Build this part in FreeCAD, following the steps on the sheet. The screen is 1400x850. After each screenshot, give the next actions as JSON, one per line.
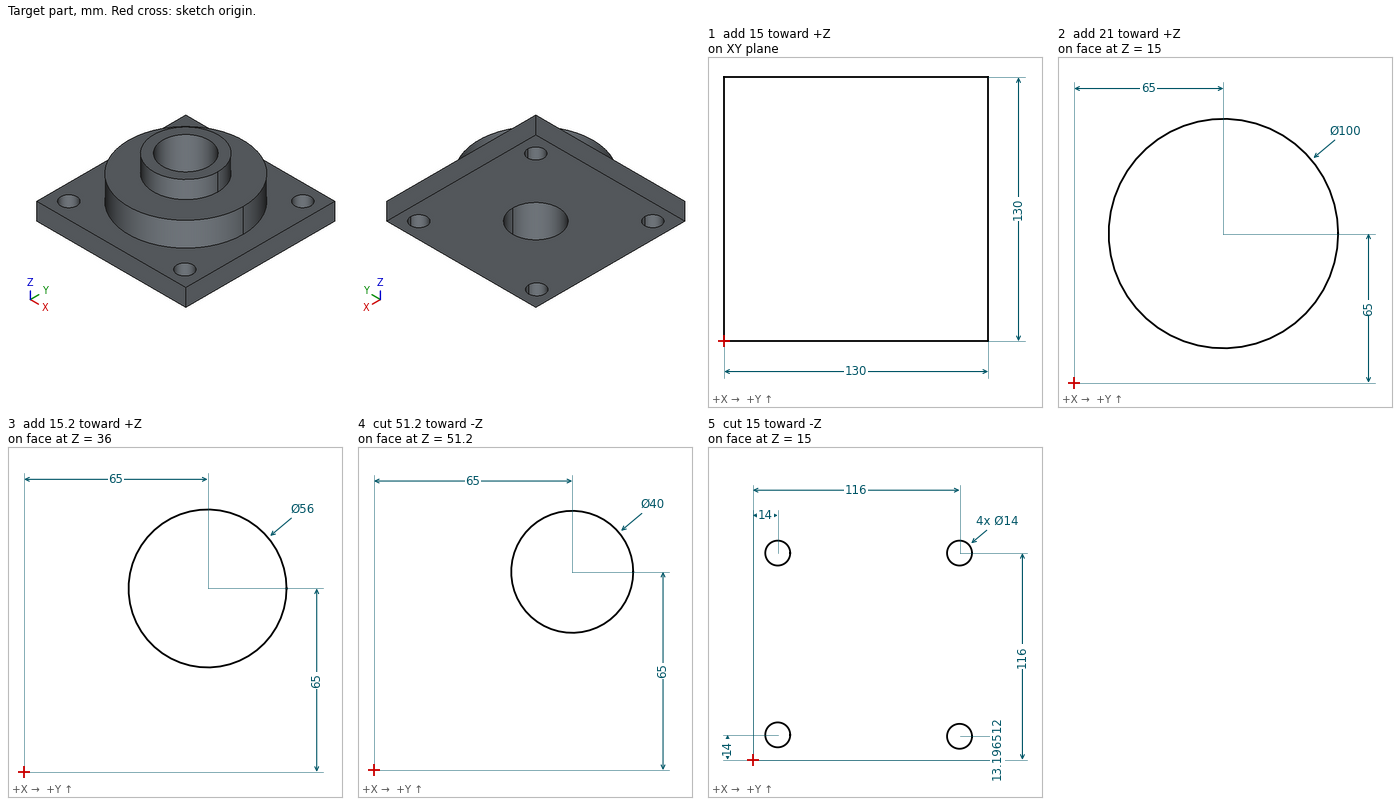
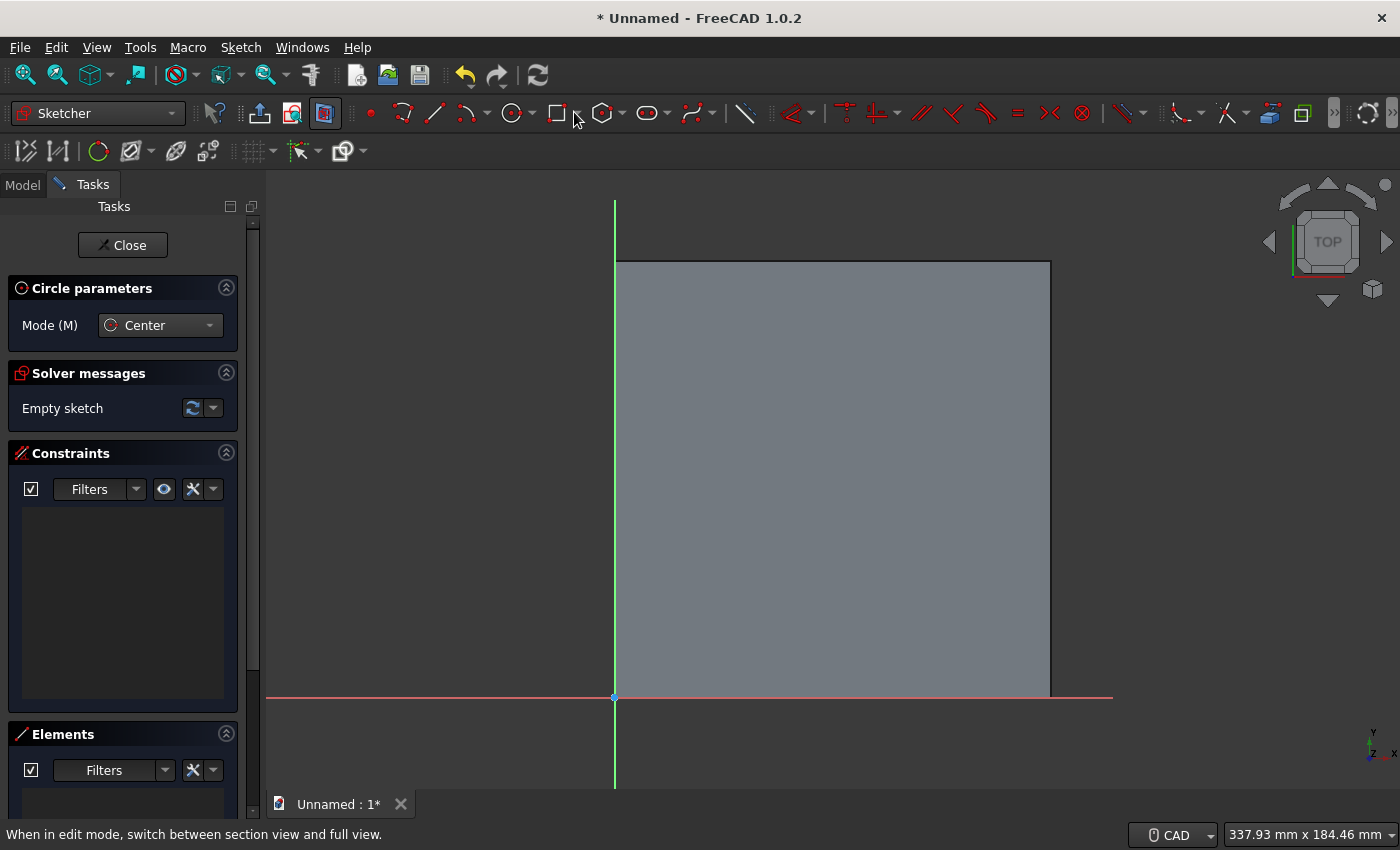
{"action": "left_click", "coordinate": [833, 480]}
{"action": "mouse_move", "coordinate": [952, 361]}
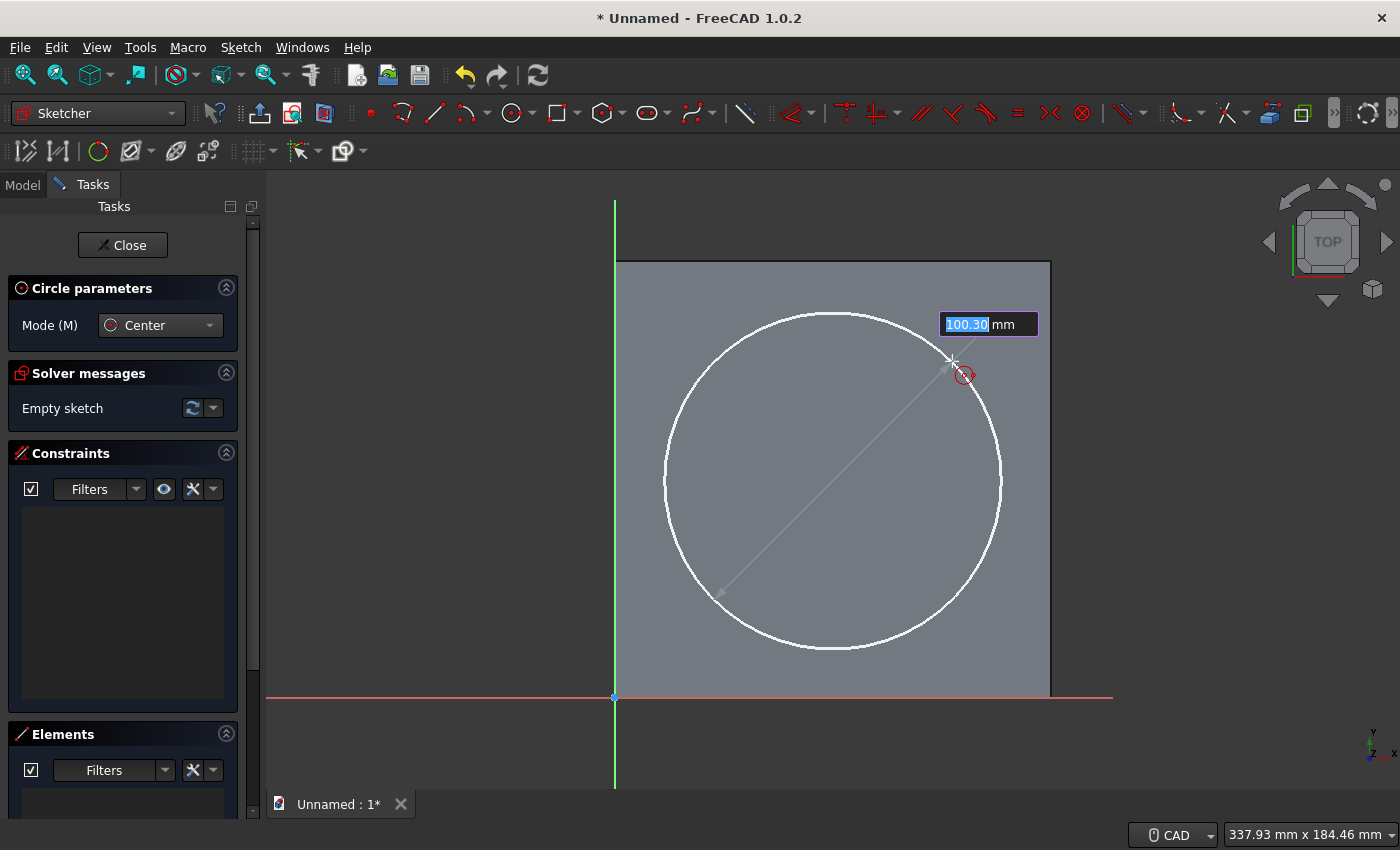
{"action": "type", "text": "100"}
{"action": "key", "text": "Return"}
{"action": "key", "text": "Escape"}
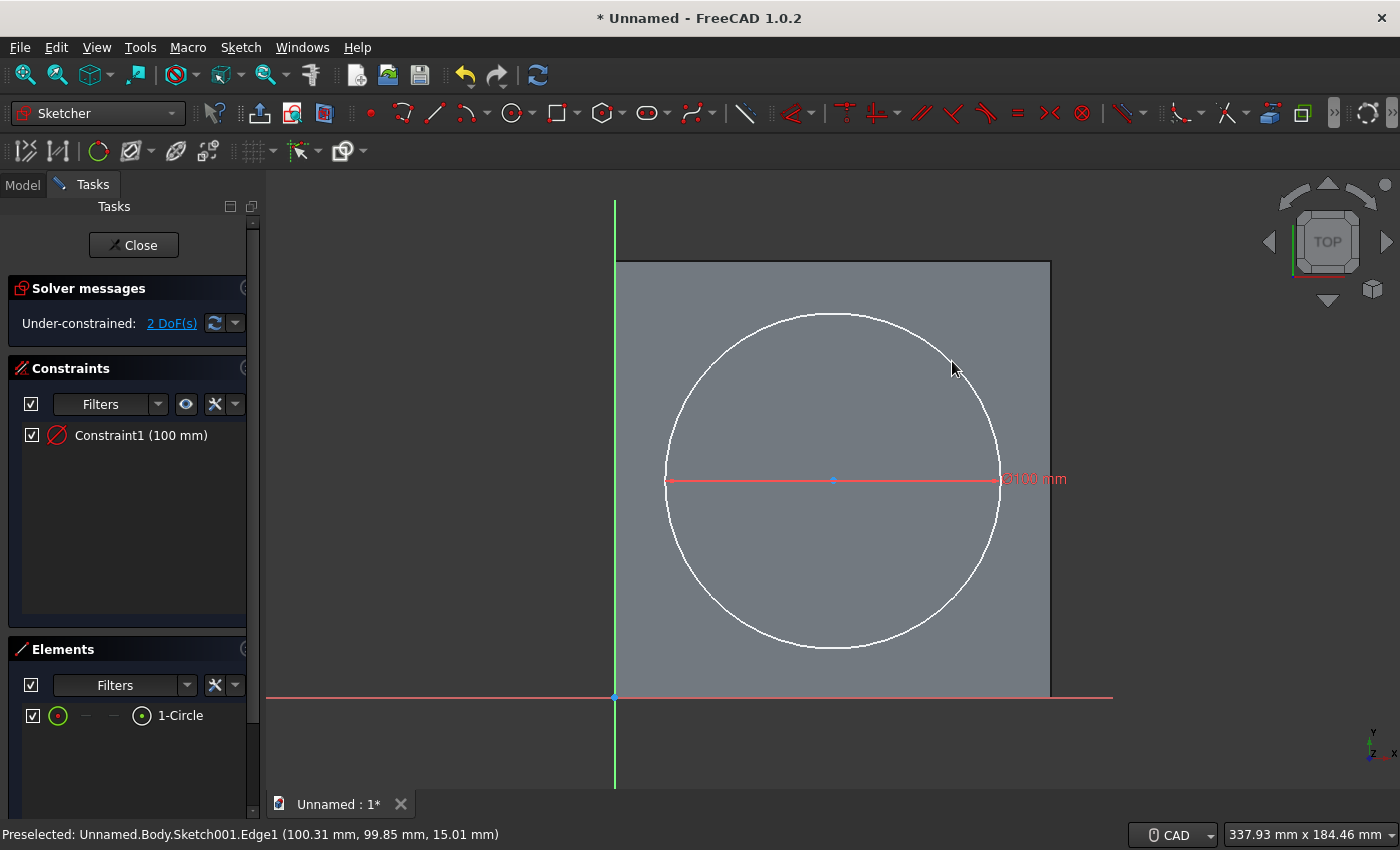
{"action": "key", "text": "d"}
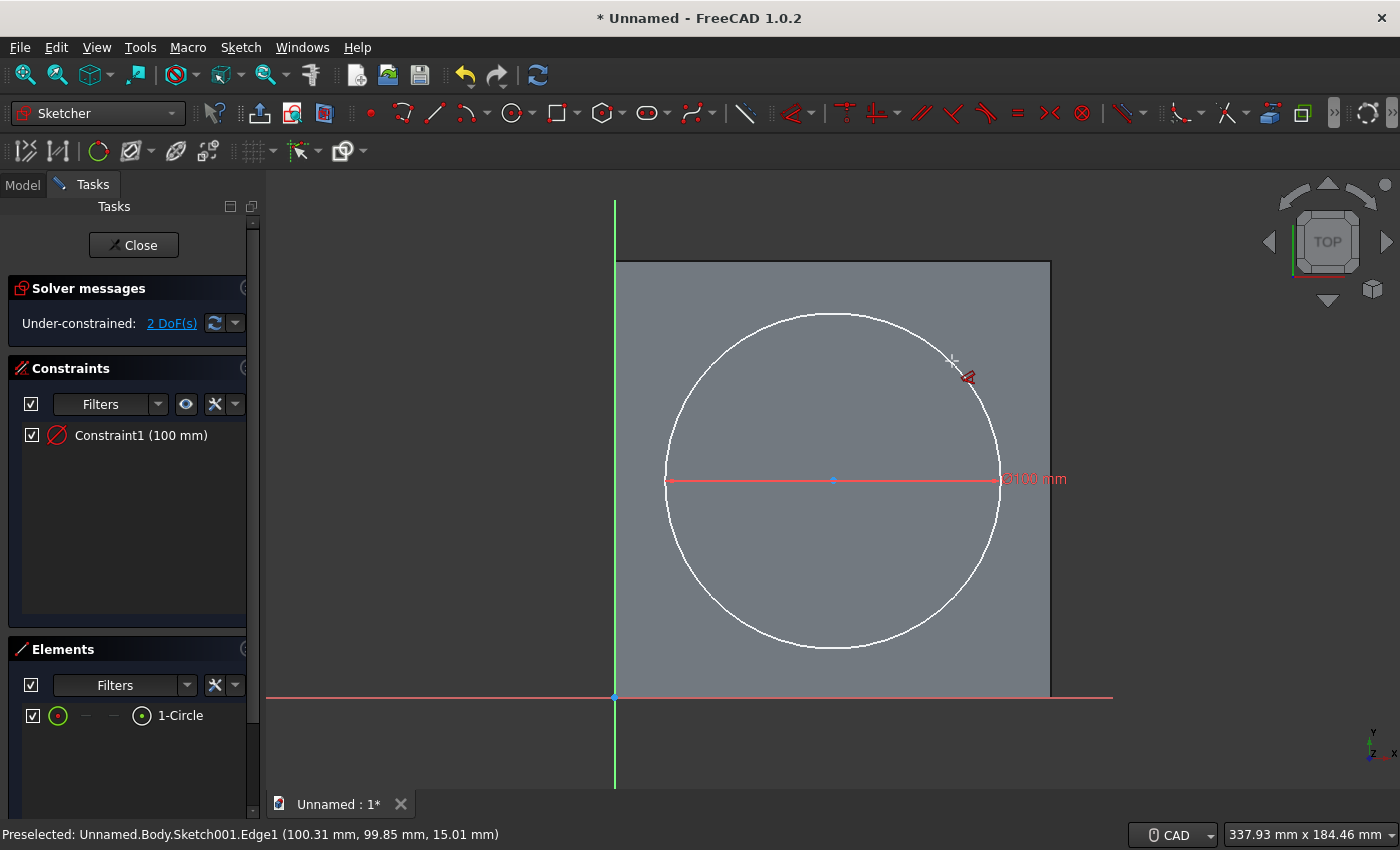
{"action": "left_click", "coordinate": [833, 481]}
{"action": "left_click", "coordinate": [724, 732]}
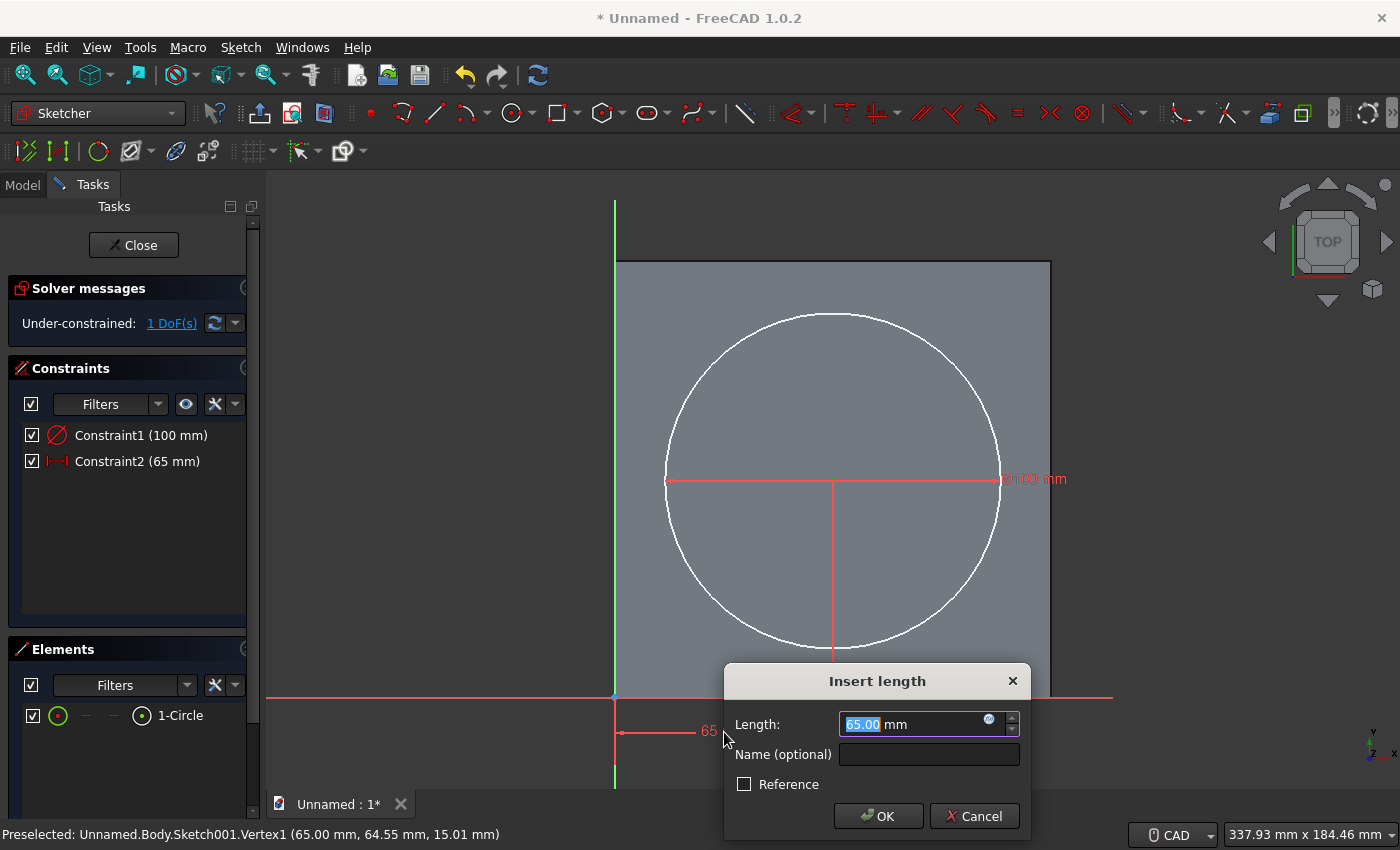
{"action": "type", "text": "65"}
{"action": "key", "text": "Return"}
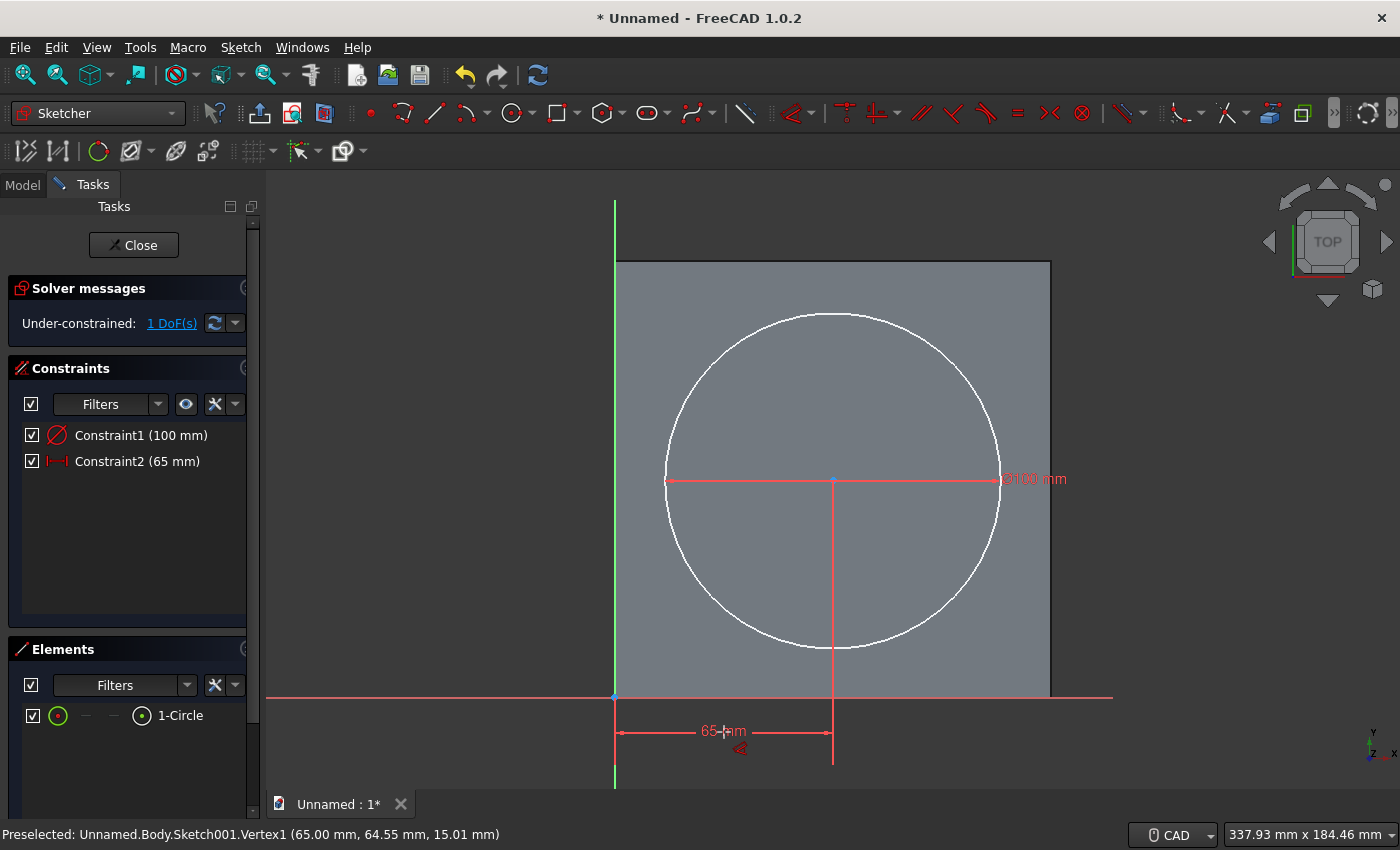
{"action": "left_click", "coordinate": [833, 481]}
{"action": "left_click", "coordinate": [581, 589]}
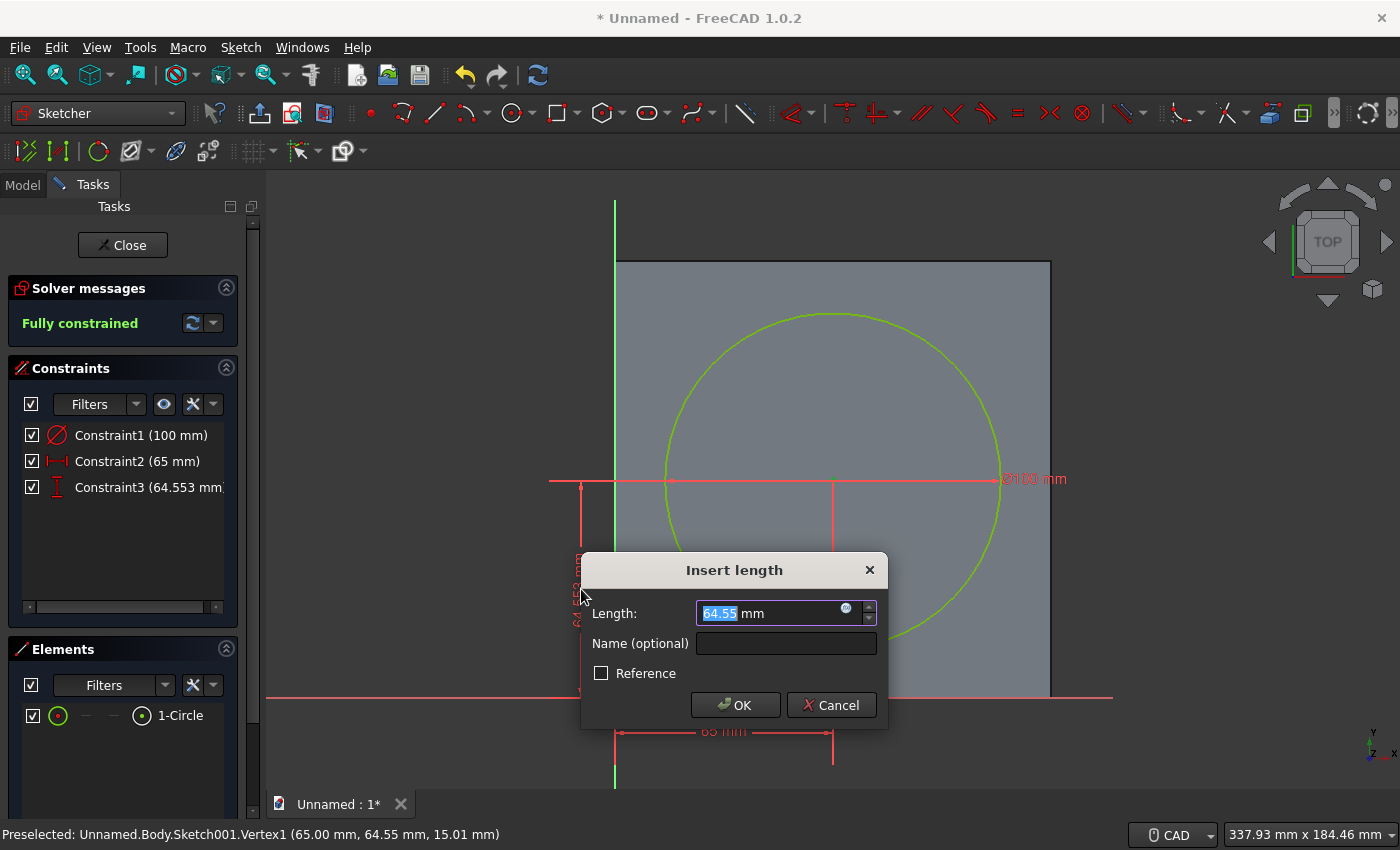
{"action": "type", "text": "65"}
{"action": "key", "text": "Return"}
{"action": "key", "text": "Escape"}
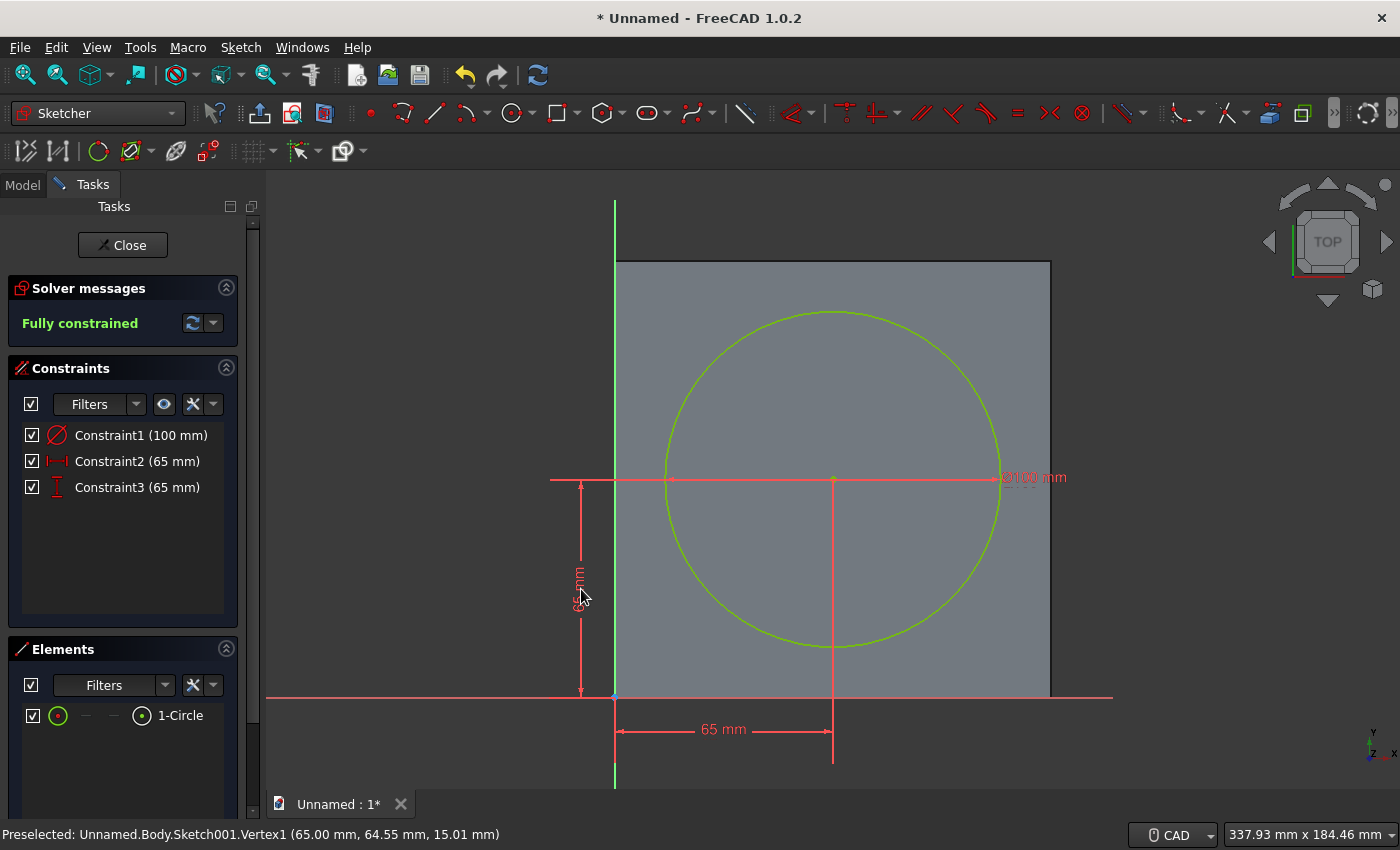
{"action": "left_click", "coordinate": [123, 245]}